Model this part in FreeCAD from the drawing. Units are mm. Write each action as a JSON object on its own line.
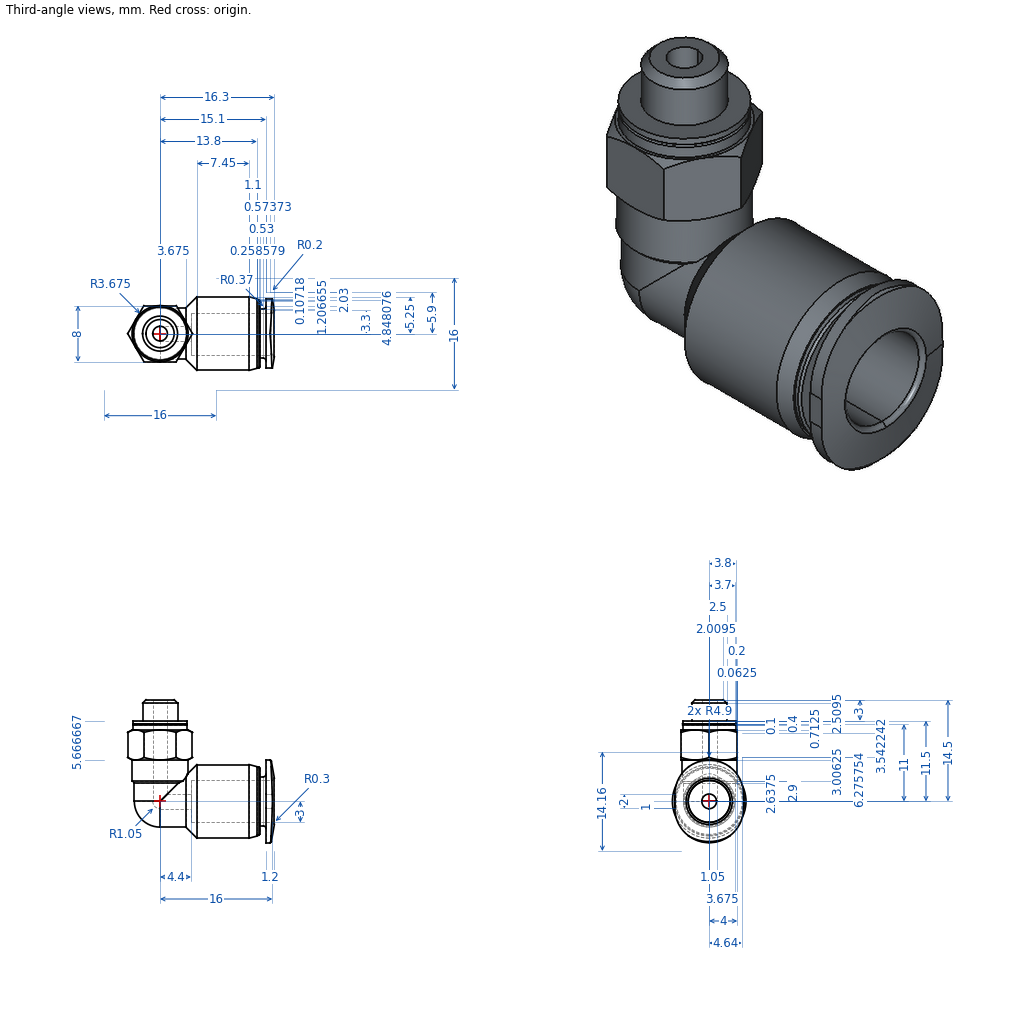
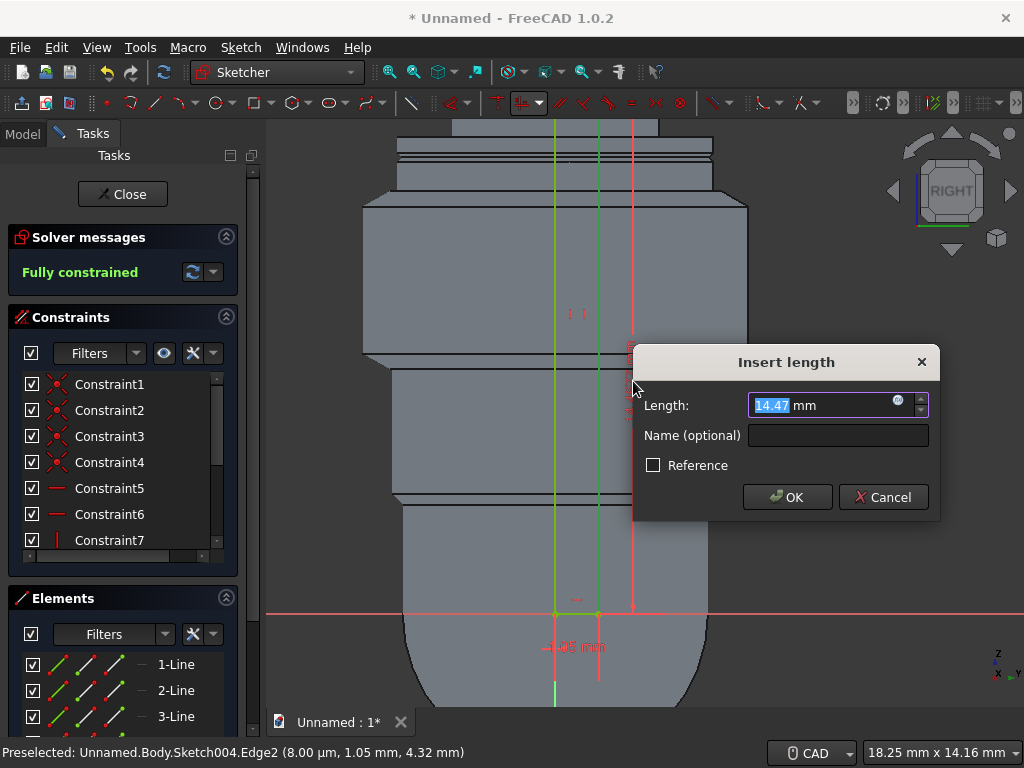
{"action": "type", "text": "14.5"}
{"action": "key", "text": "Return"}
{"action": "key", "text": "Escape"}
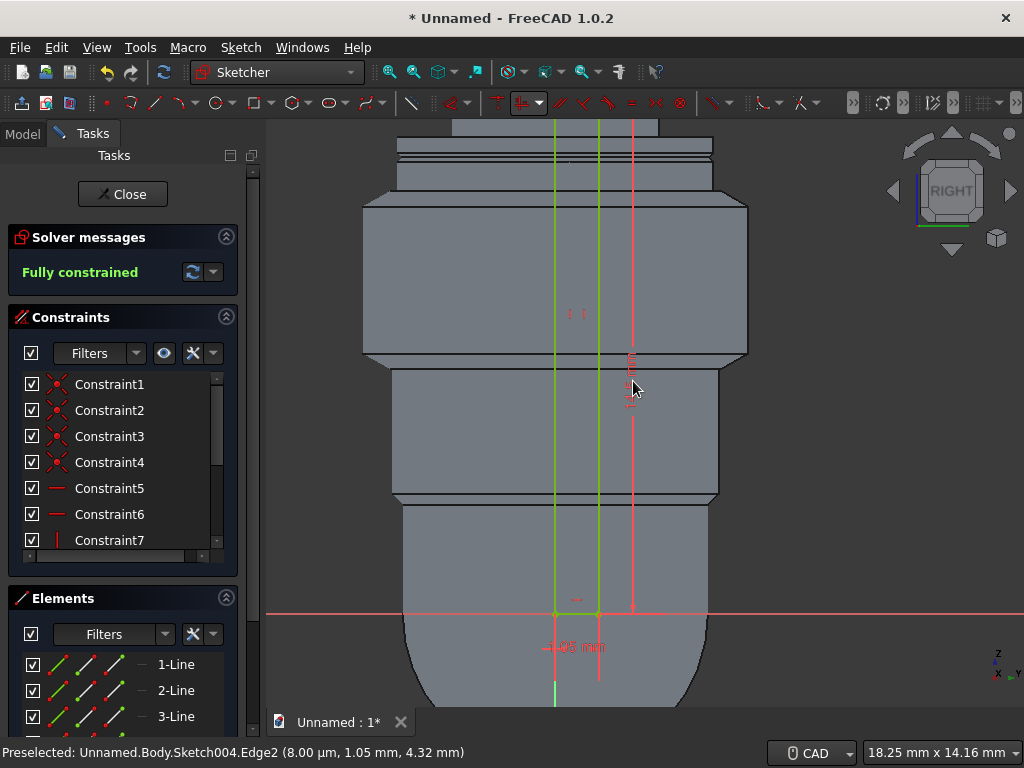
{"action": "left_click", "coordinate": [123, 194]}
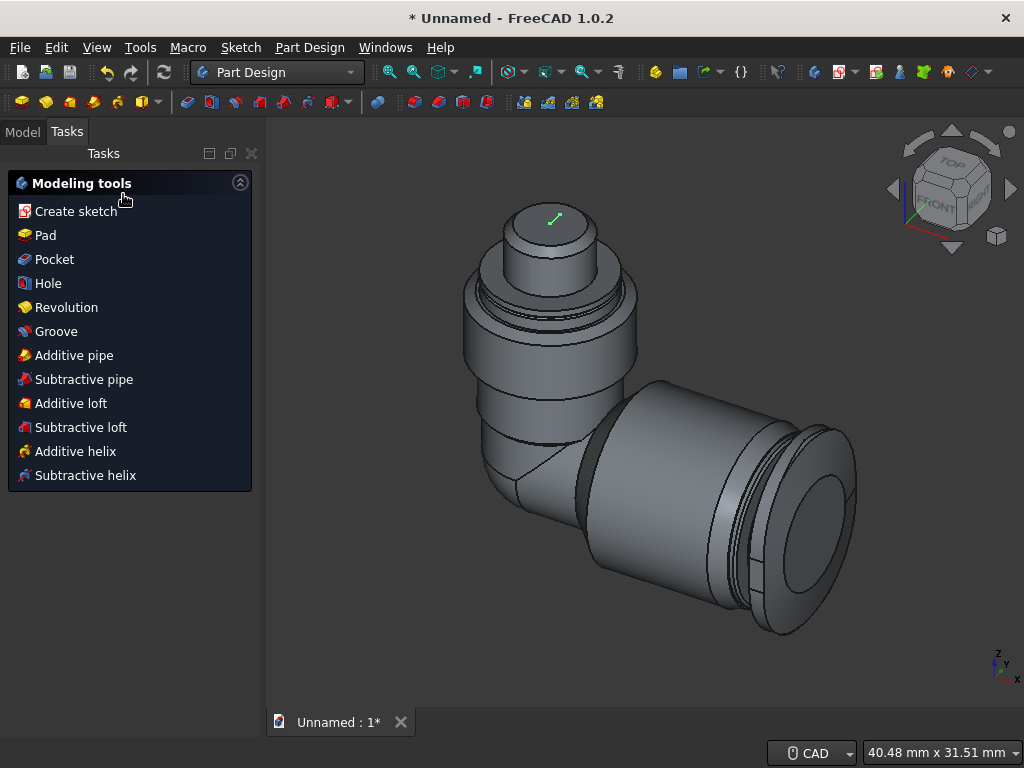
{"action": "left_click", "coordinate": [236, 102]}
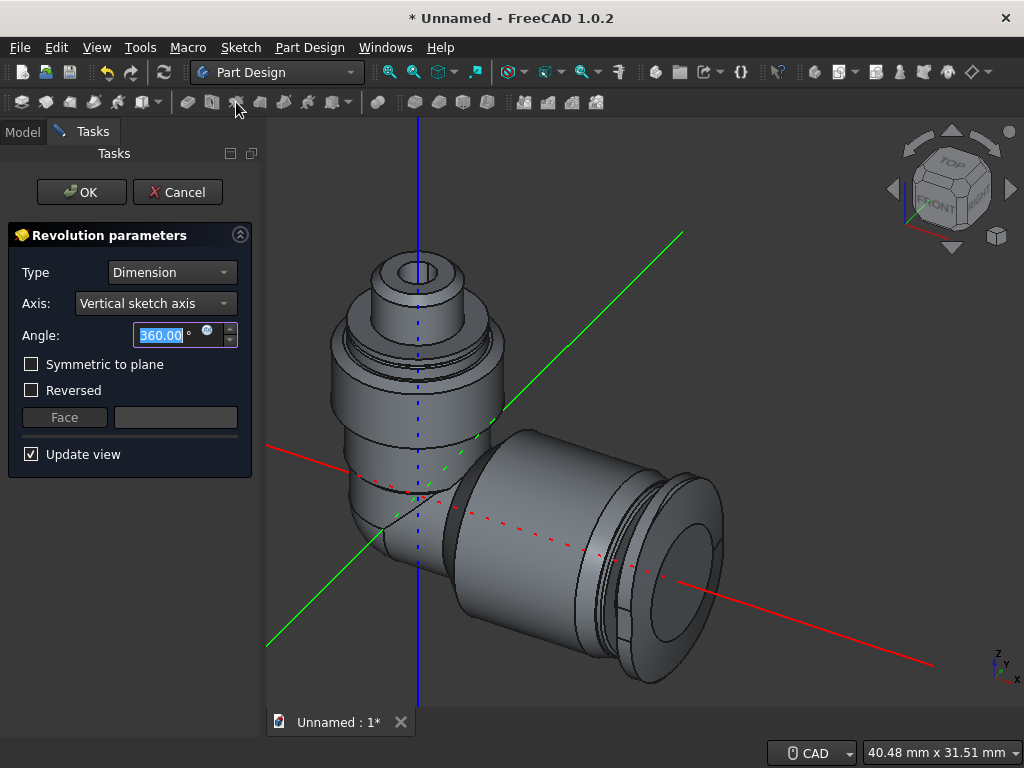
{"action": "left_click", "coordinate": [82, 192]}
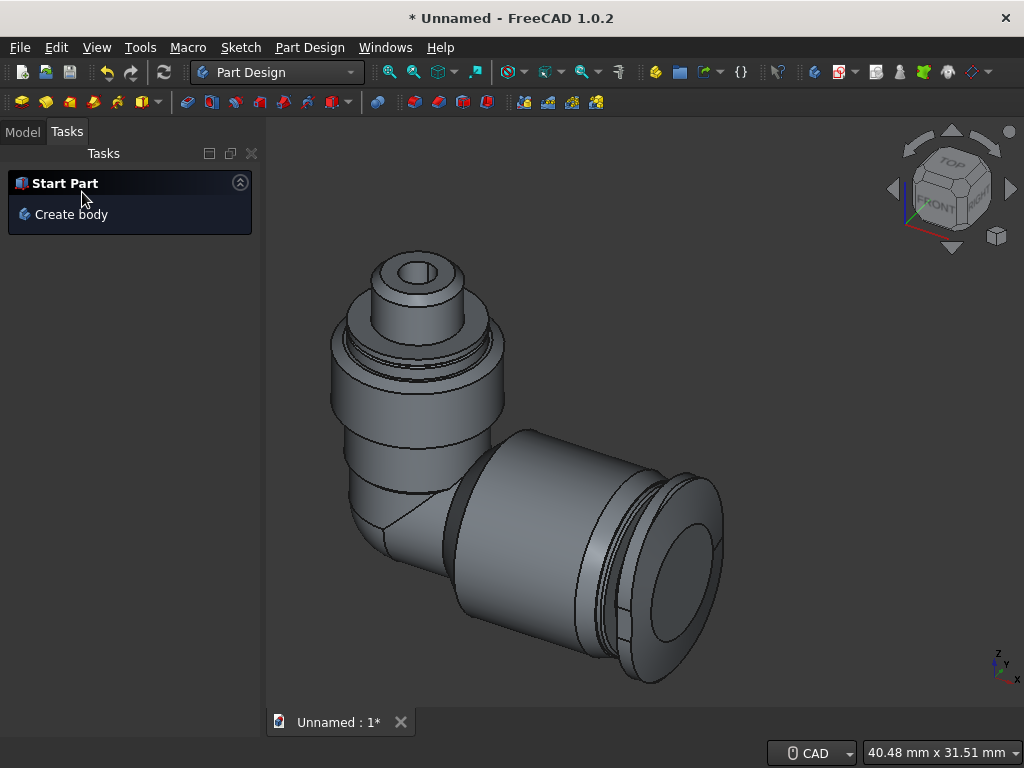
{"action": "left_click", "coordinate": [390, 72]}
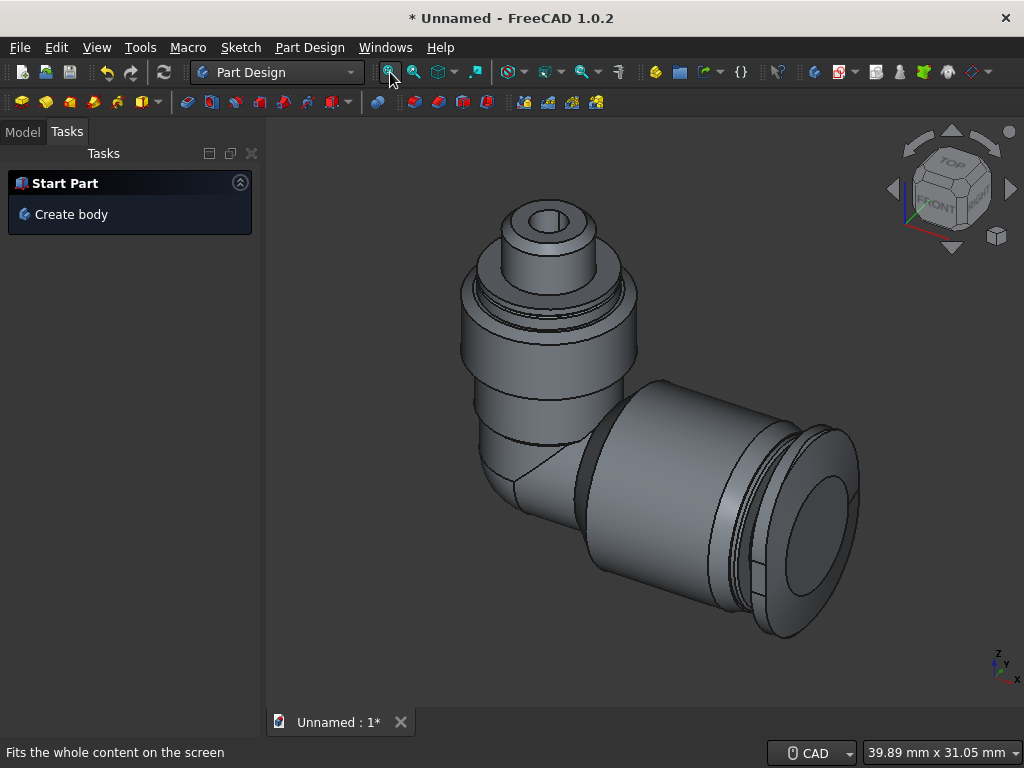
{"action": "left_click", "coordinate": [840, 72]}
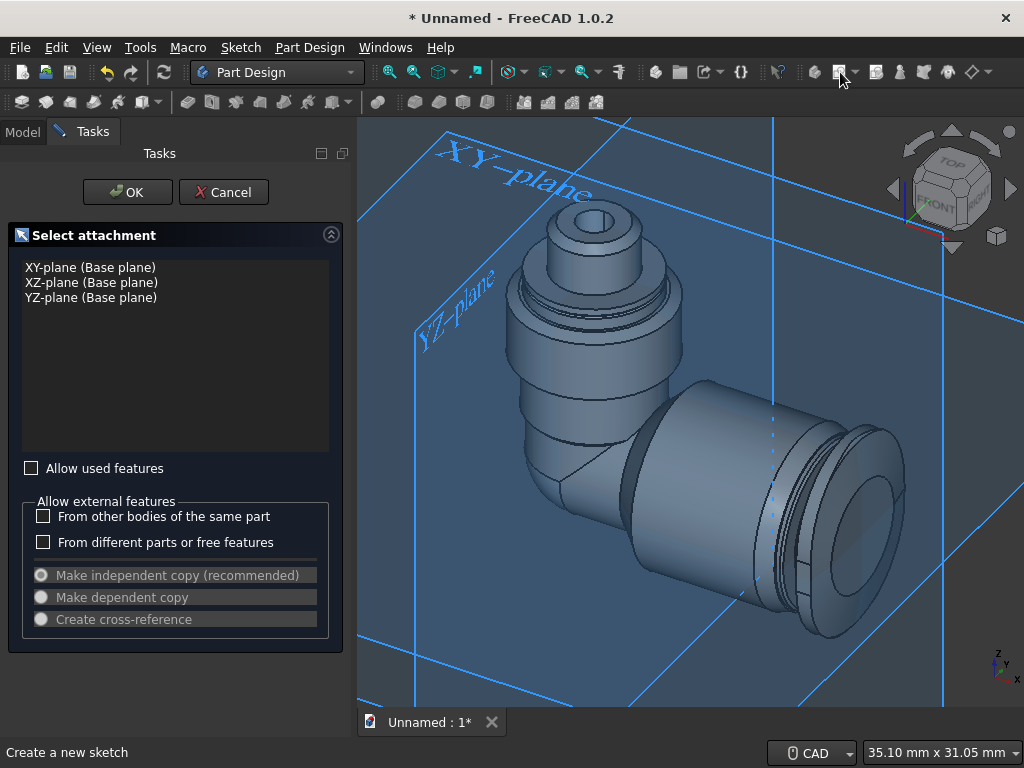
{"action": "left_click", "coordinate": [82, 282]}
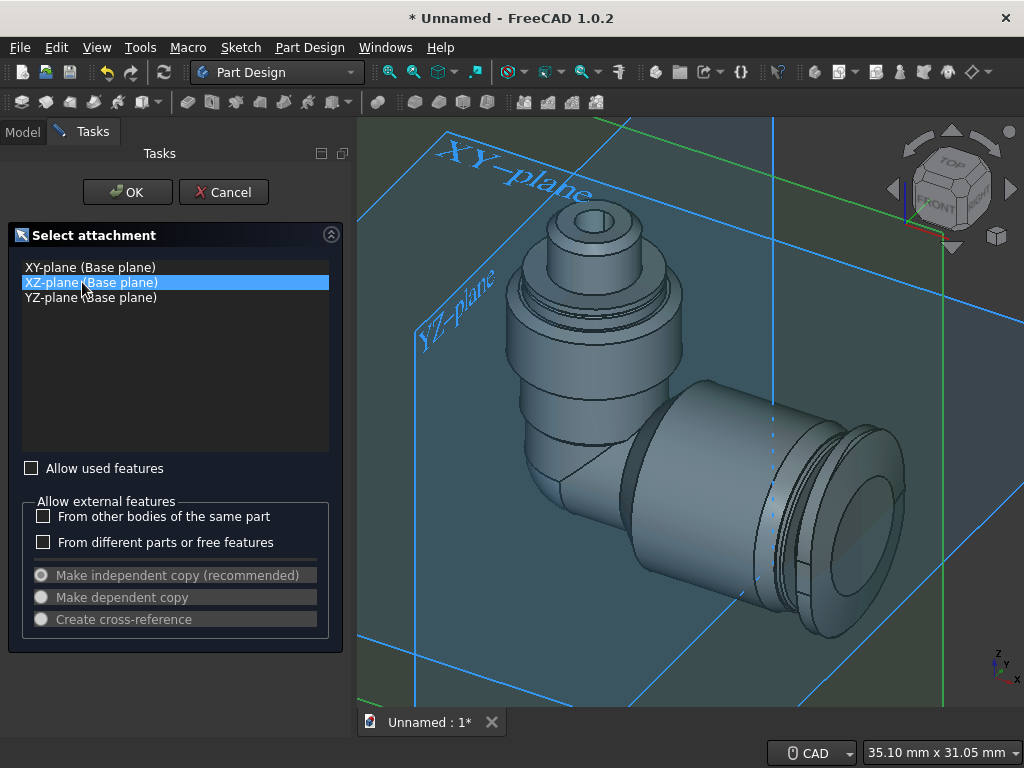
{"action": "left_click", "coordinate": [128, 192]}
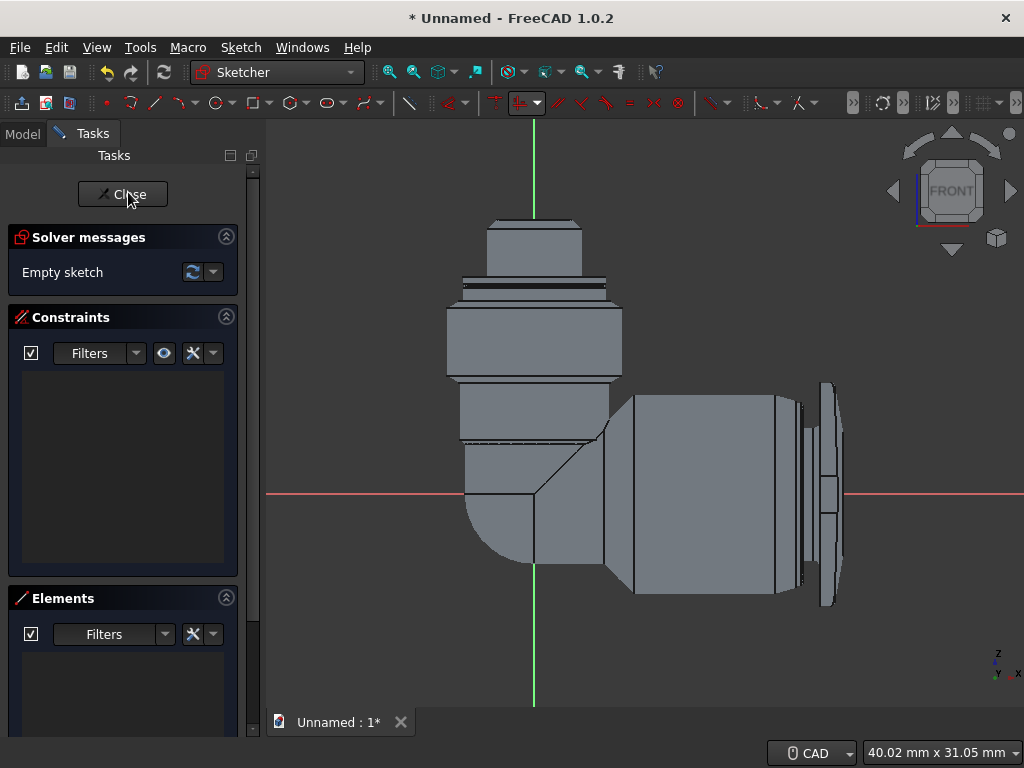
{"action": "left_click", "coordinate": [70, 104]}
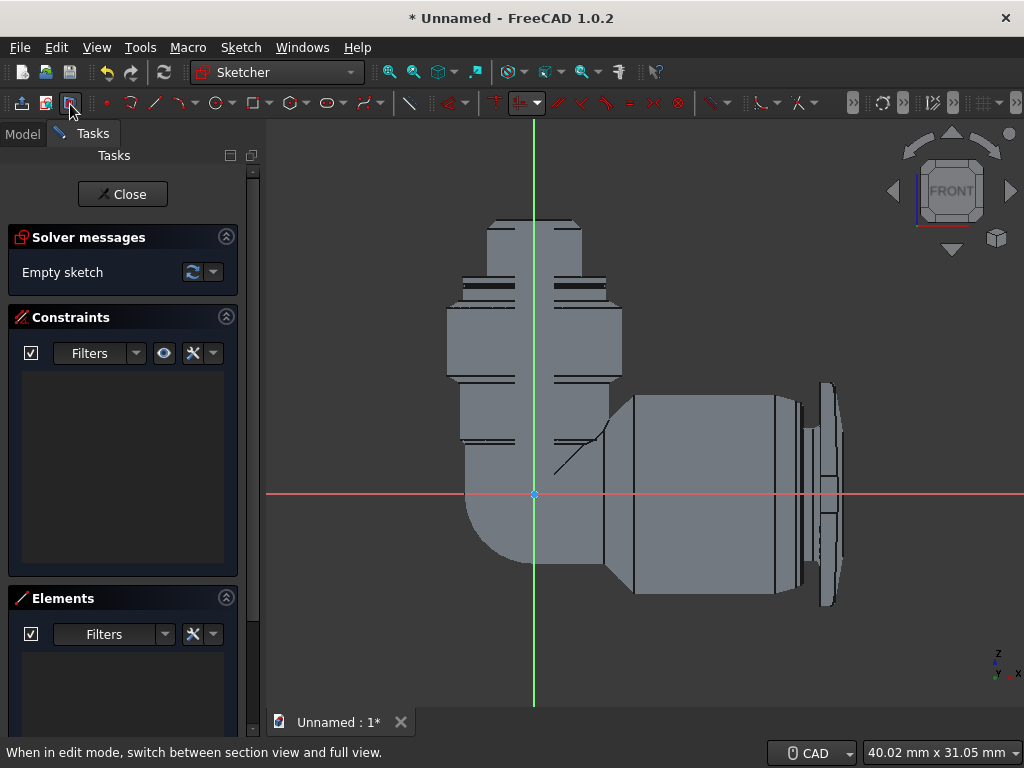
{"action": "scroll", "coordinate": [294, 147], "scroll_direction": "down", "scroll_amount": 1}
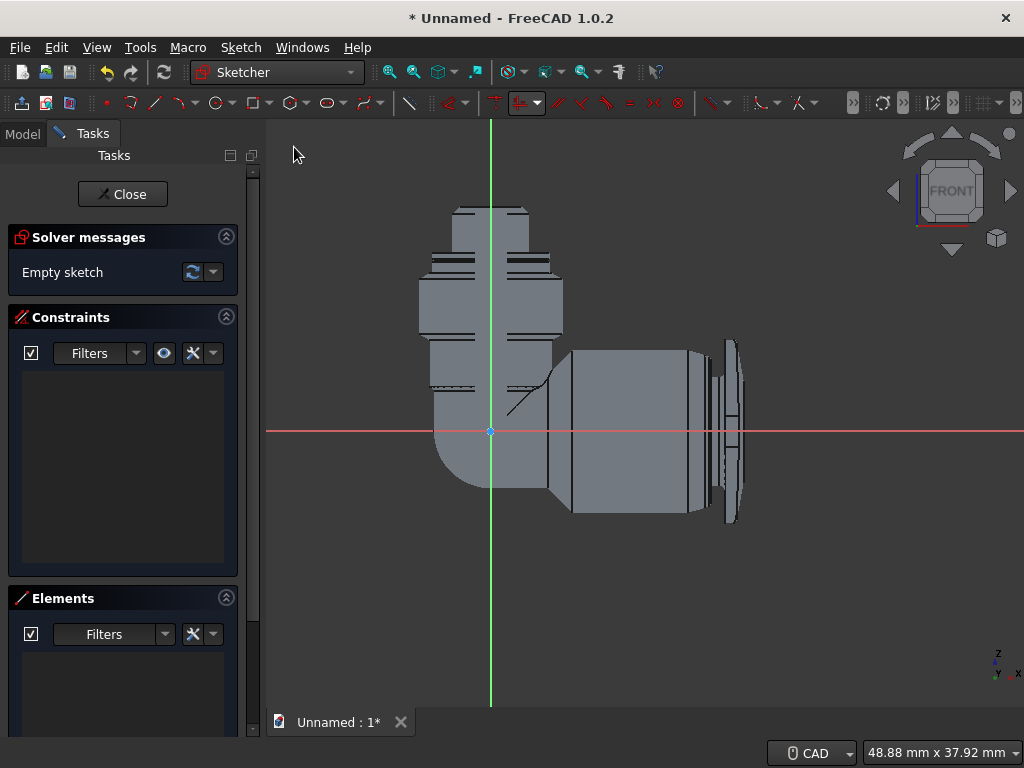
{"action": "scroll", "coordinate": [675, 547], "scroll_direction": "up", "scroll_amount": 2}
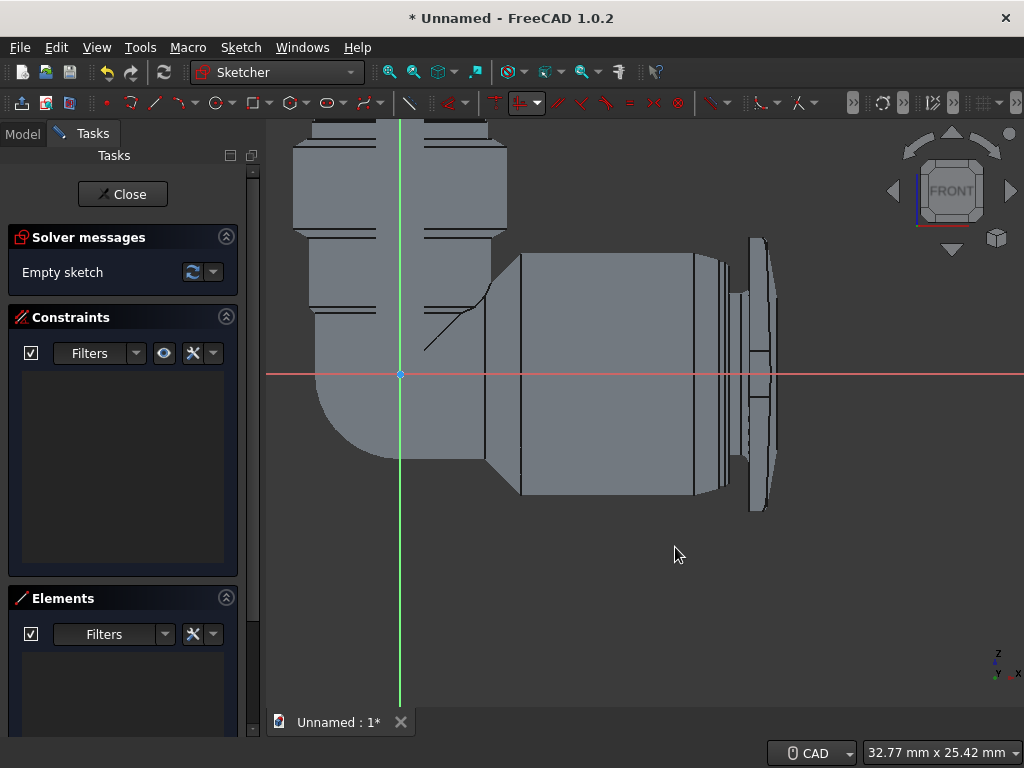
{"action": "left_click", "coordinate": [132, 104]}